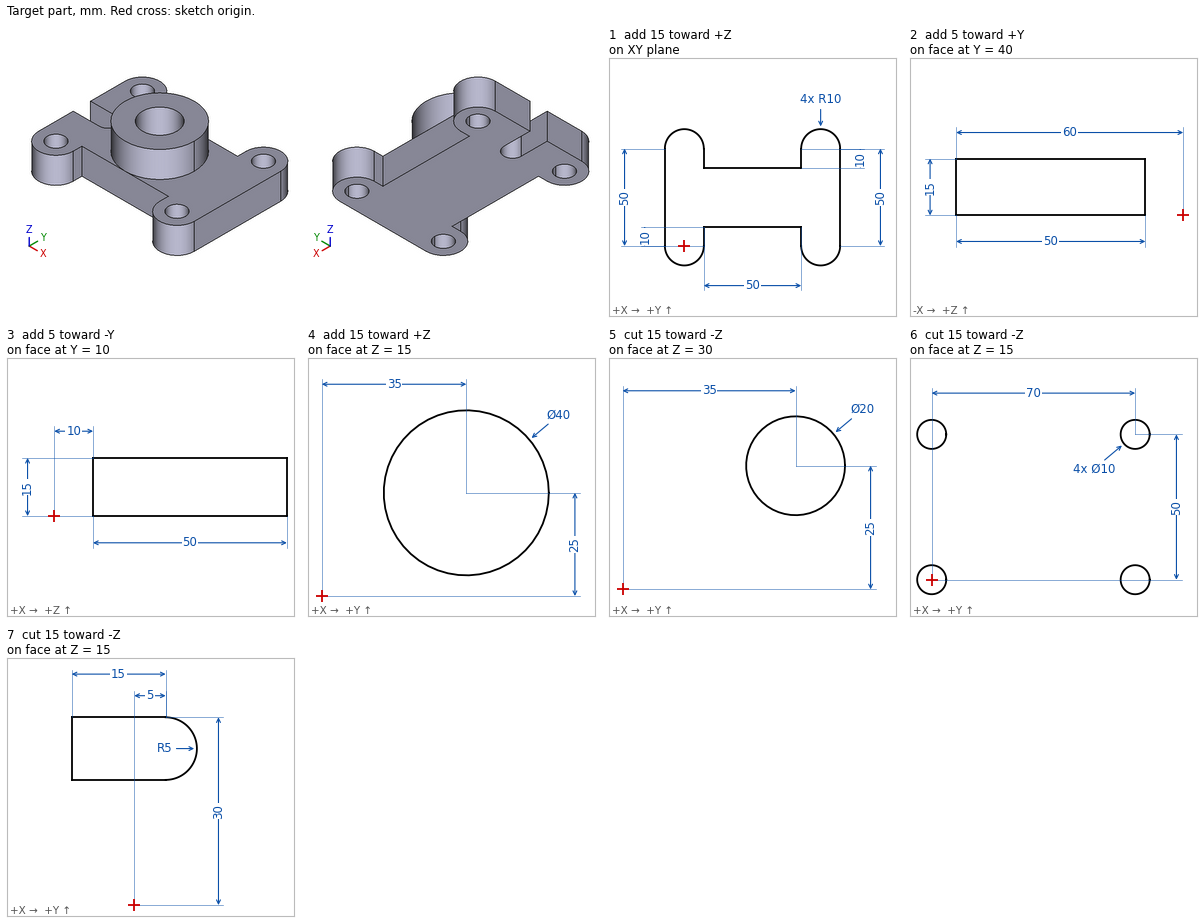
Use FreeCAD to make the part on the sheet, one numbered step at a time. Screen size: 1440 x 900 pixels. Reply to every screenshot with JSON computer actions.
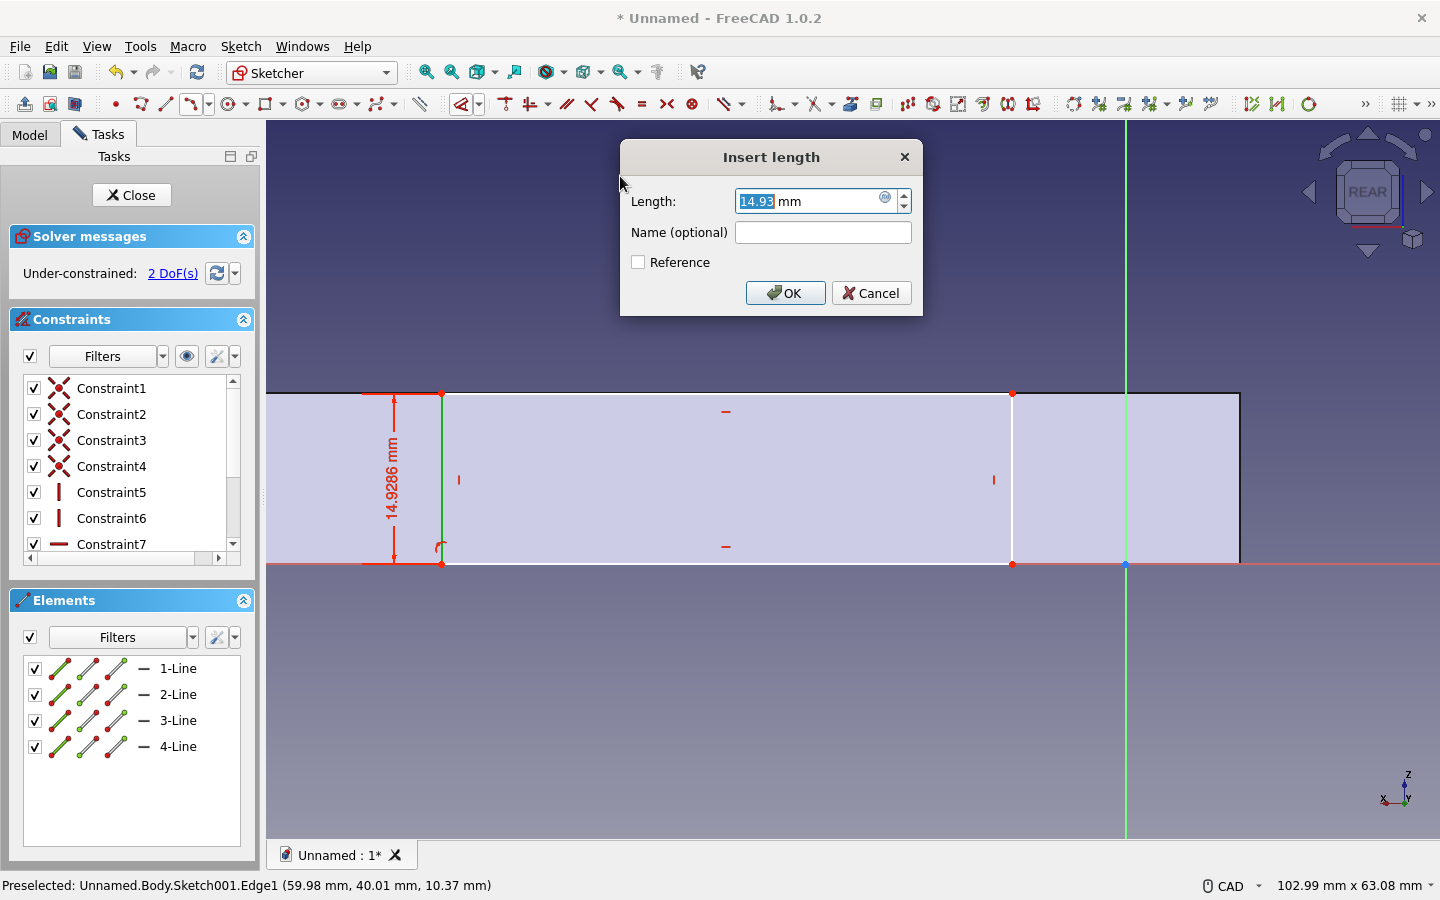
{"action": "type", "text": "15"}
{"action": "key", "text": "Return"}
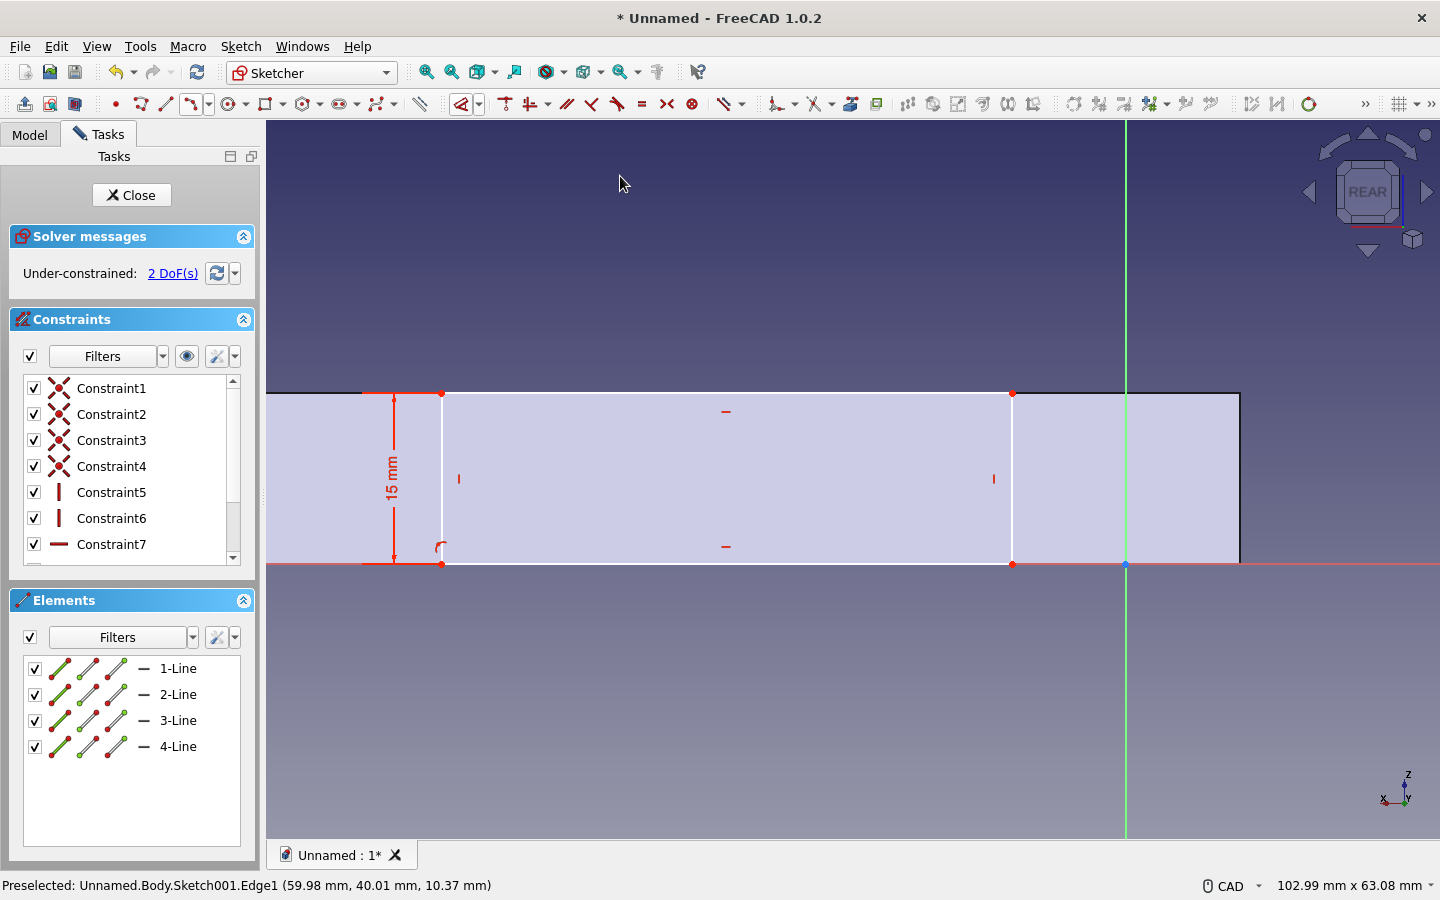
{"action": "left_click", "coordinate": [613, 564]}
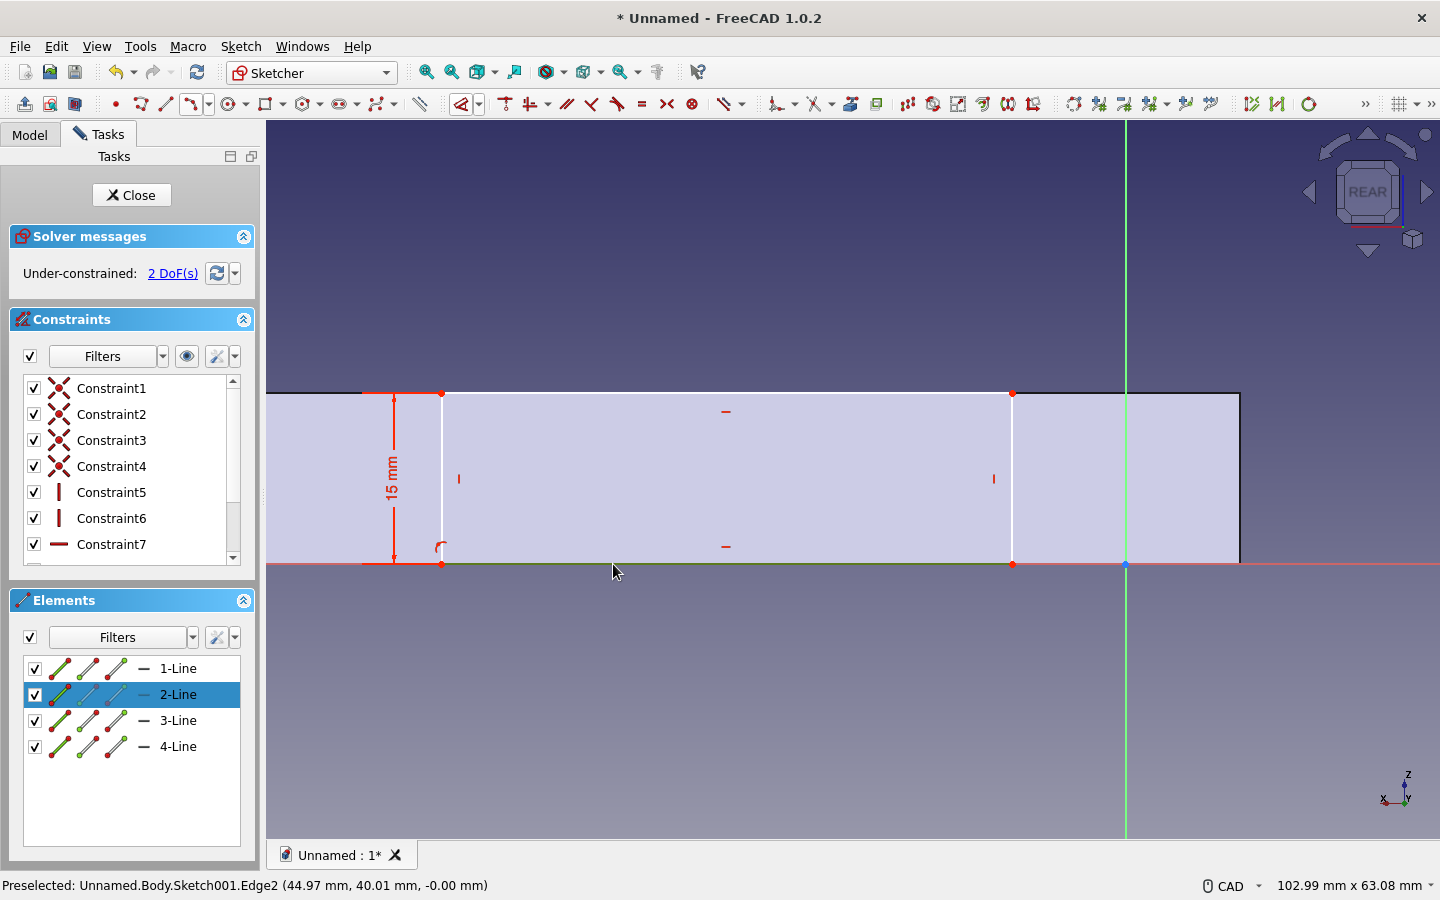
{"action": "key", "text": "l"}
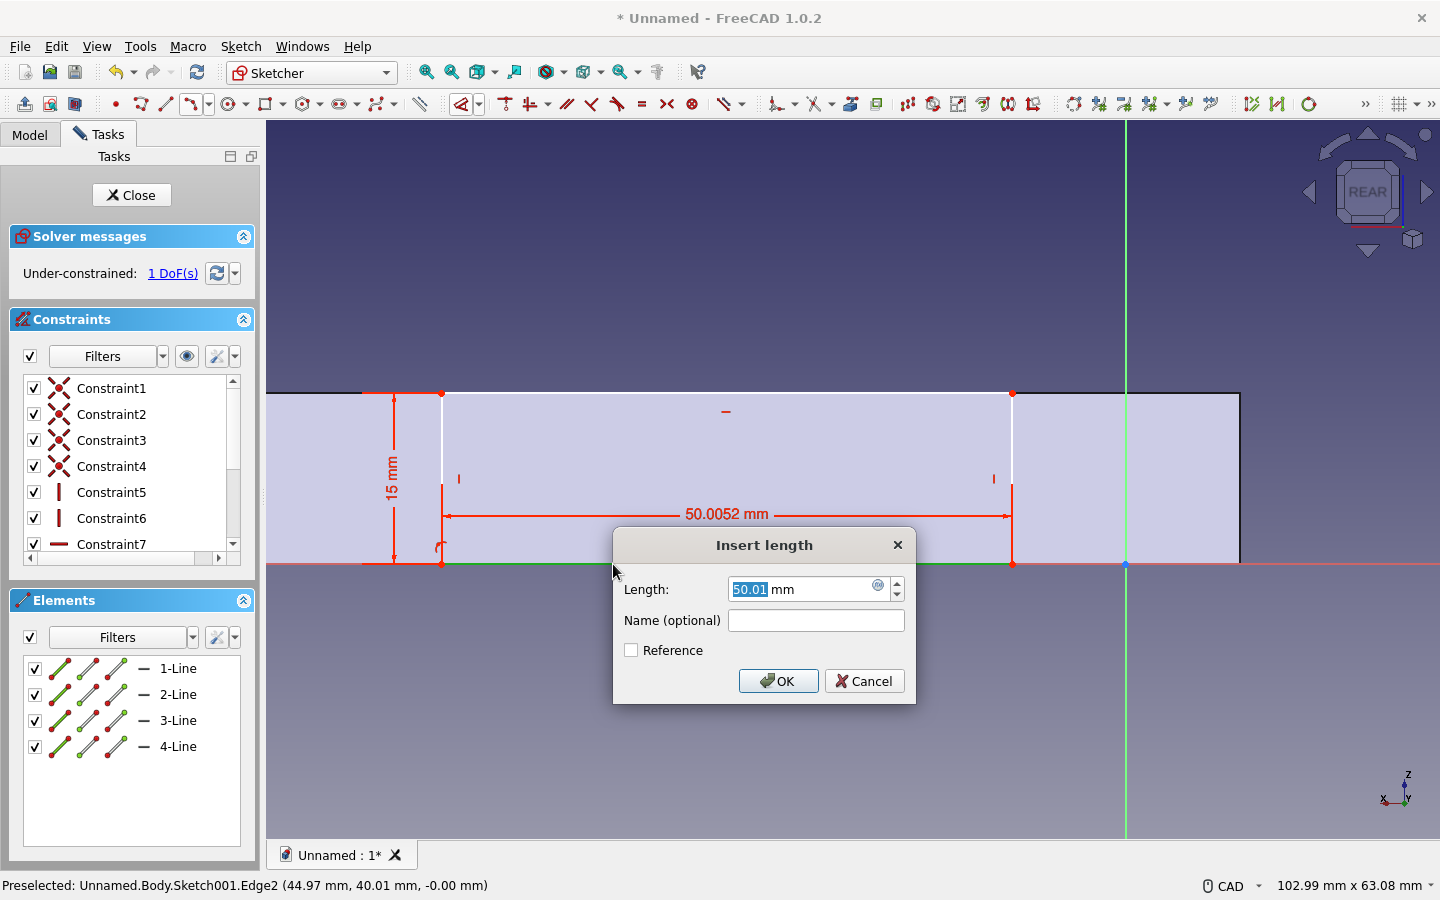
{"action": "type", "text": "50"}
{"action": "key", "text": "Return"}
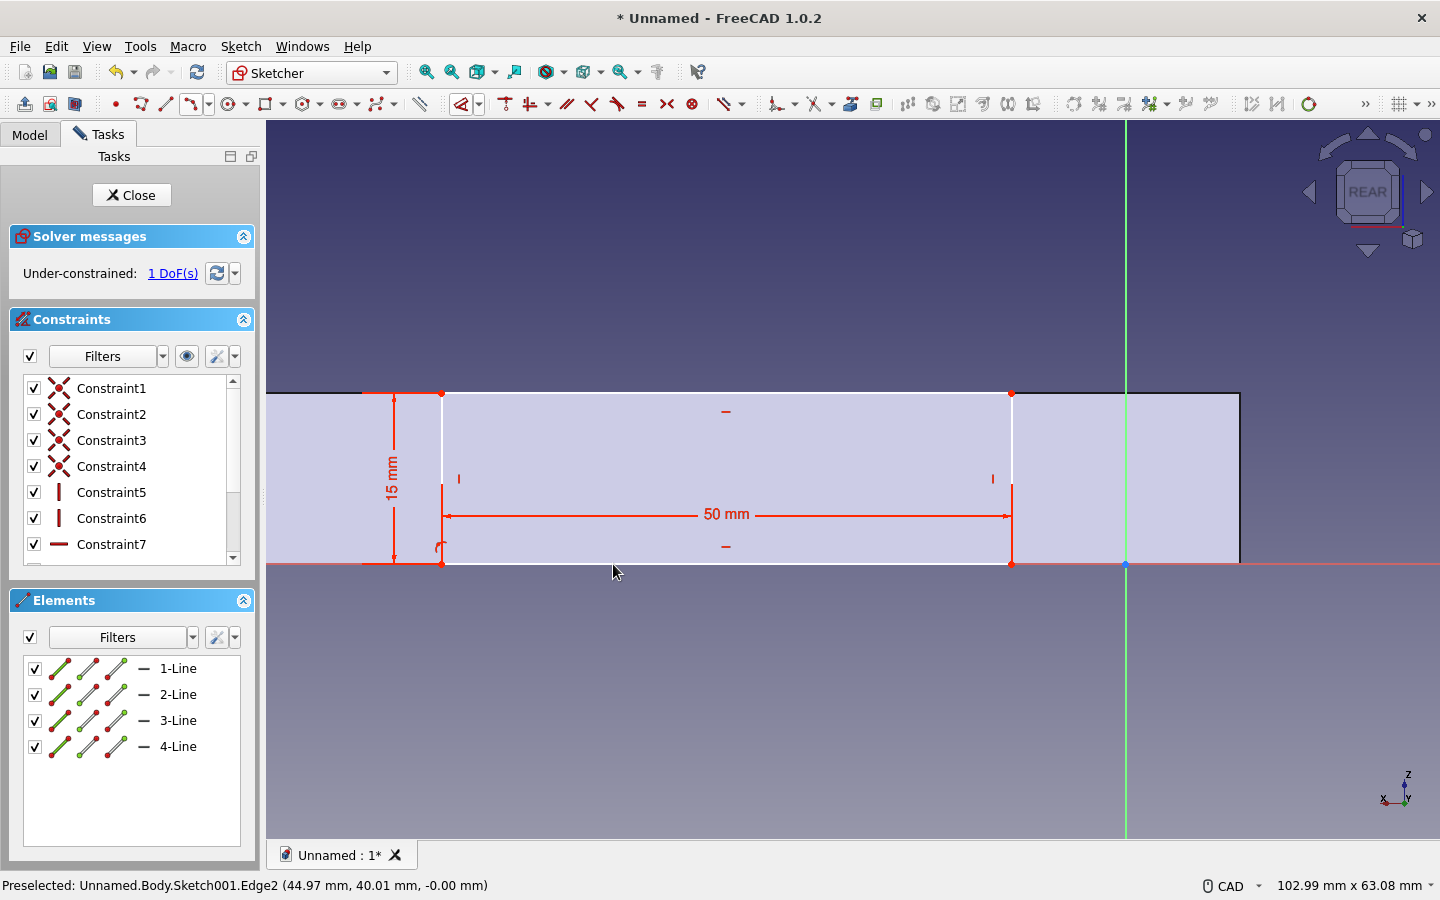
{"action": "left_click", "coordinate": [442, 393]}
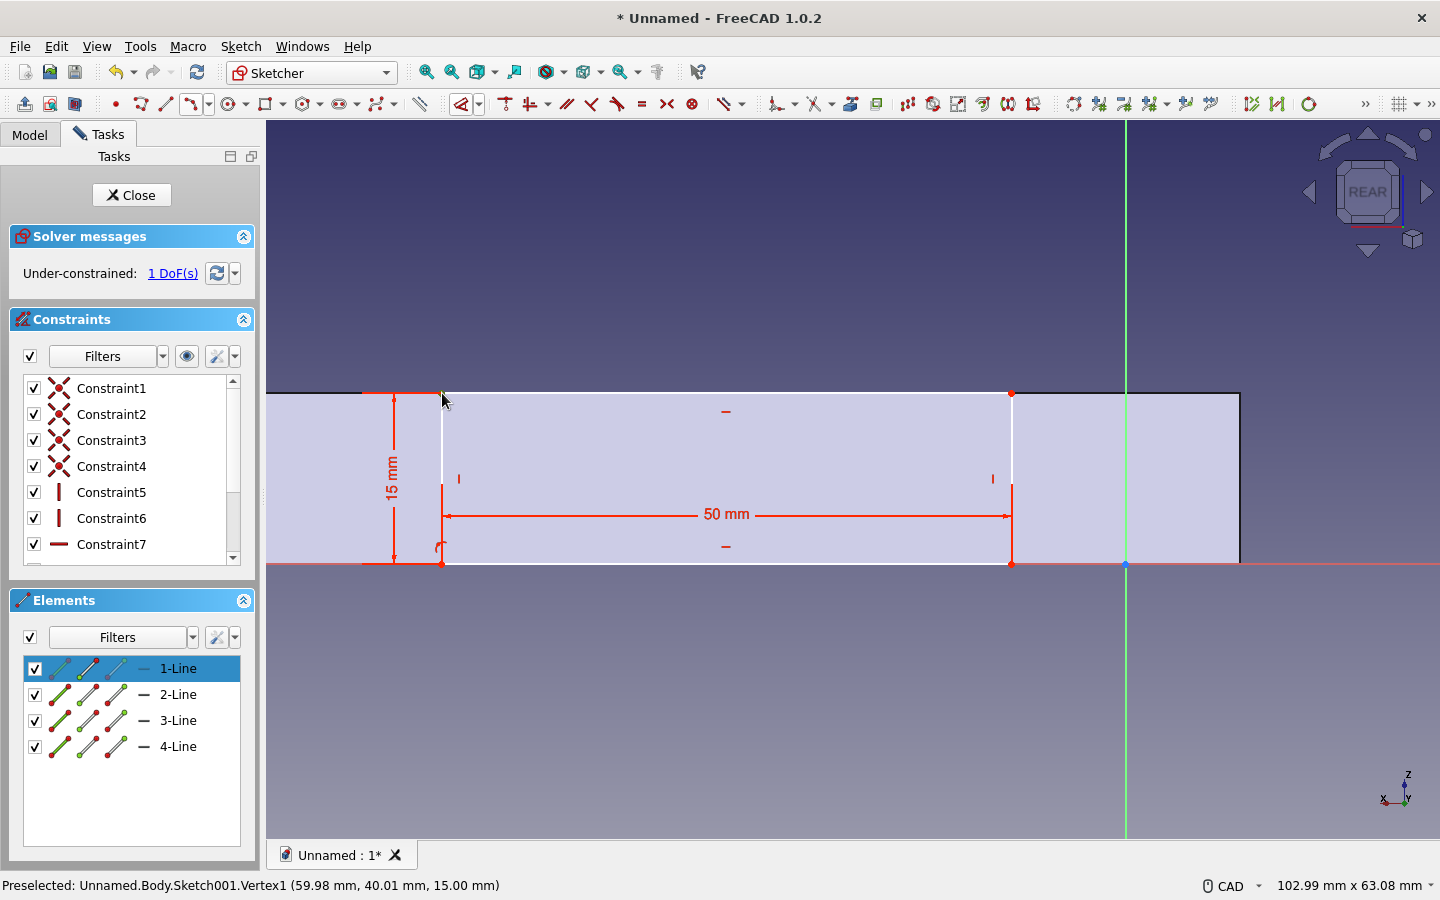
{"action": "left_click", "coordinate": [478, 104]}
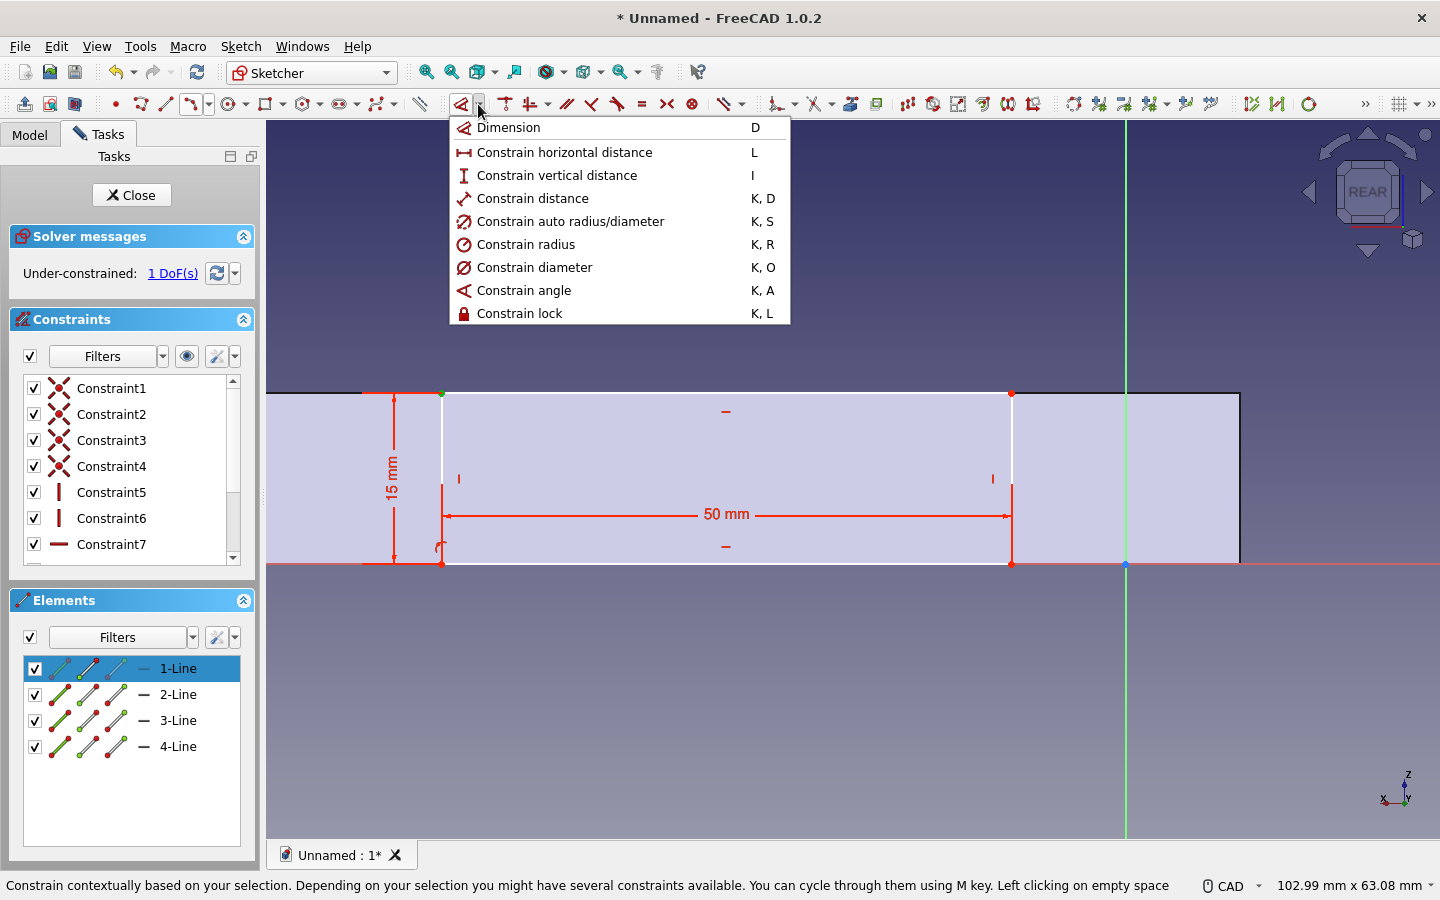
{"action": "left_click", "coordinate": [620, 152]}